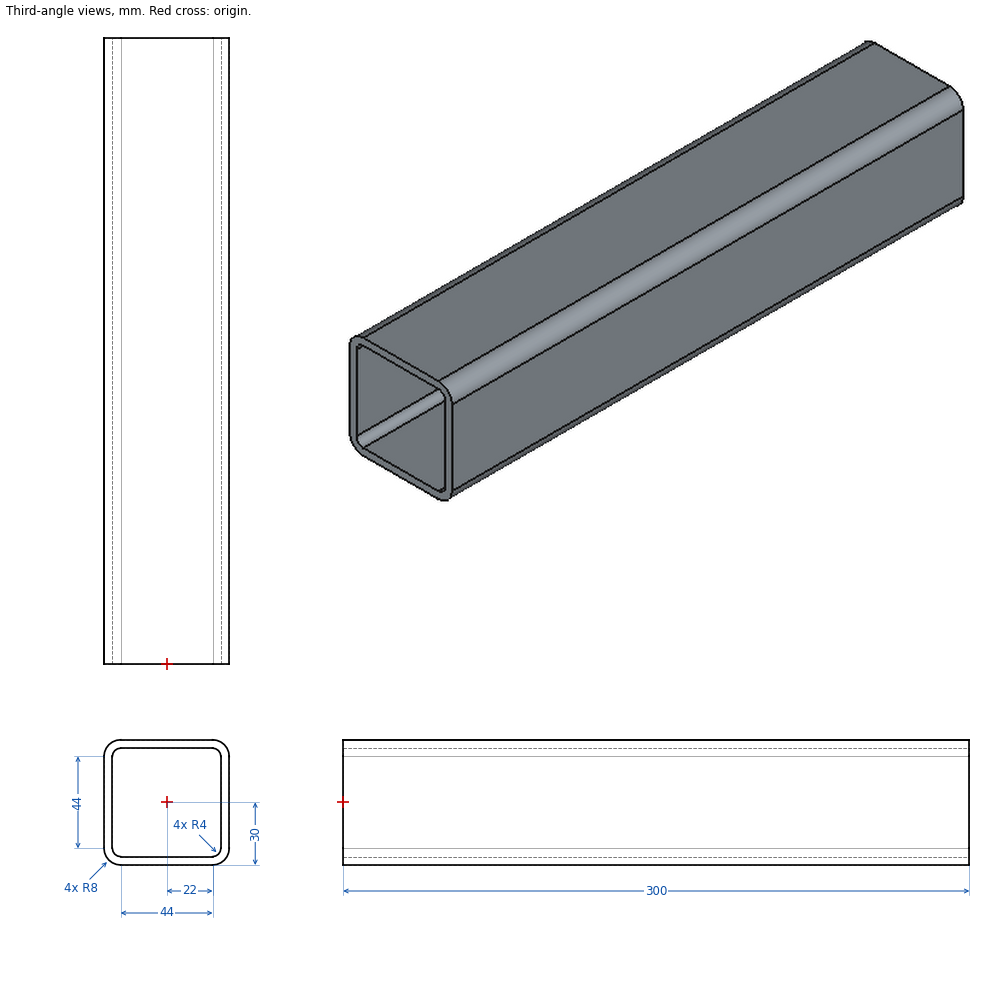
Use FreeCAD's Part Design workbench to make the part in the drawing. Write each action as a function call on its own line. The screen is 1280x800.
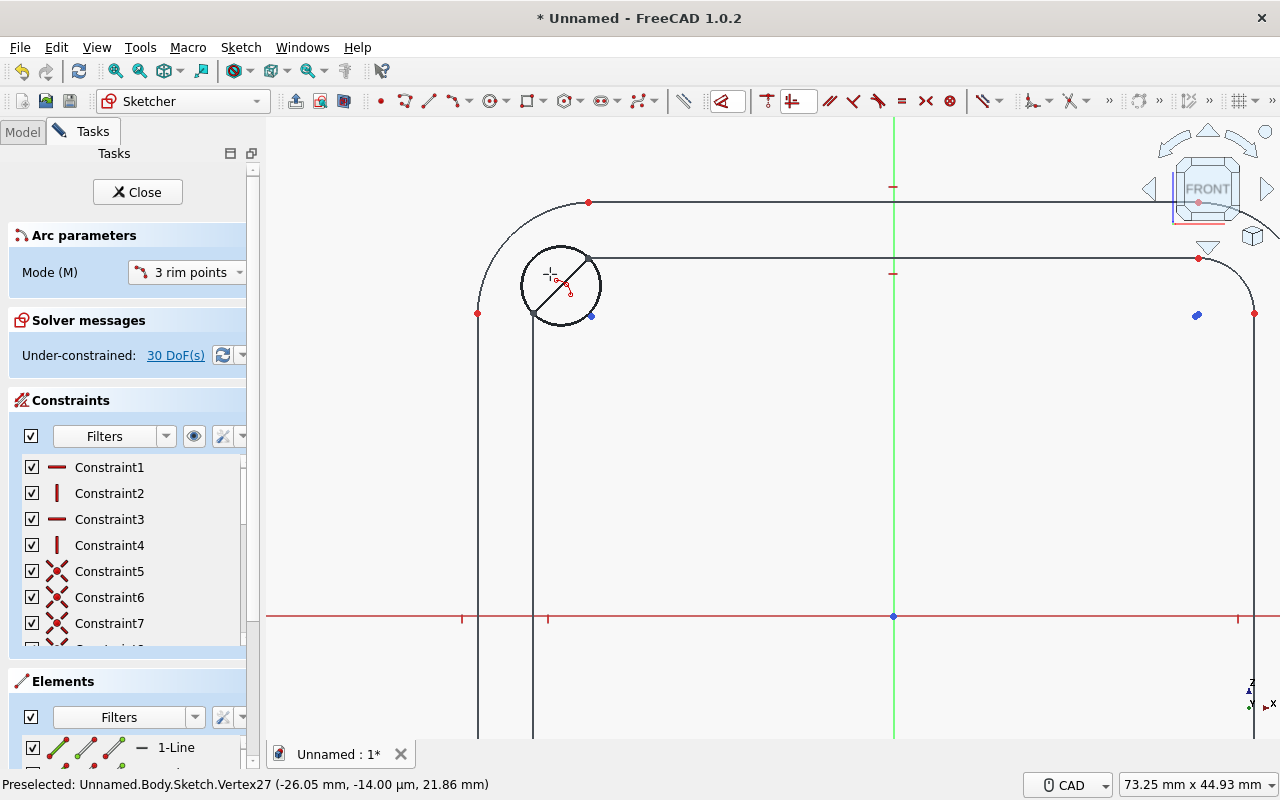
click(550, 273)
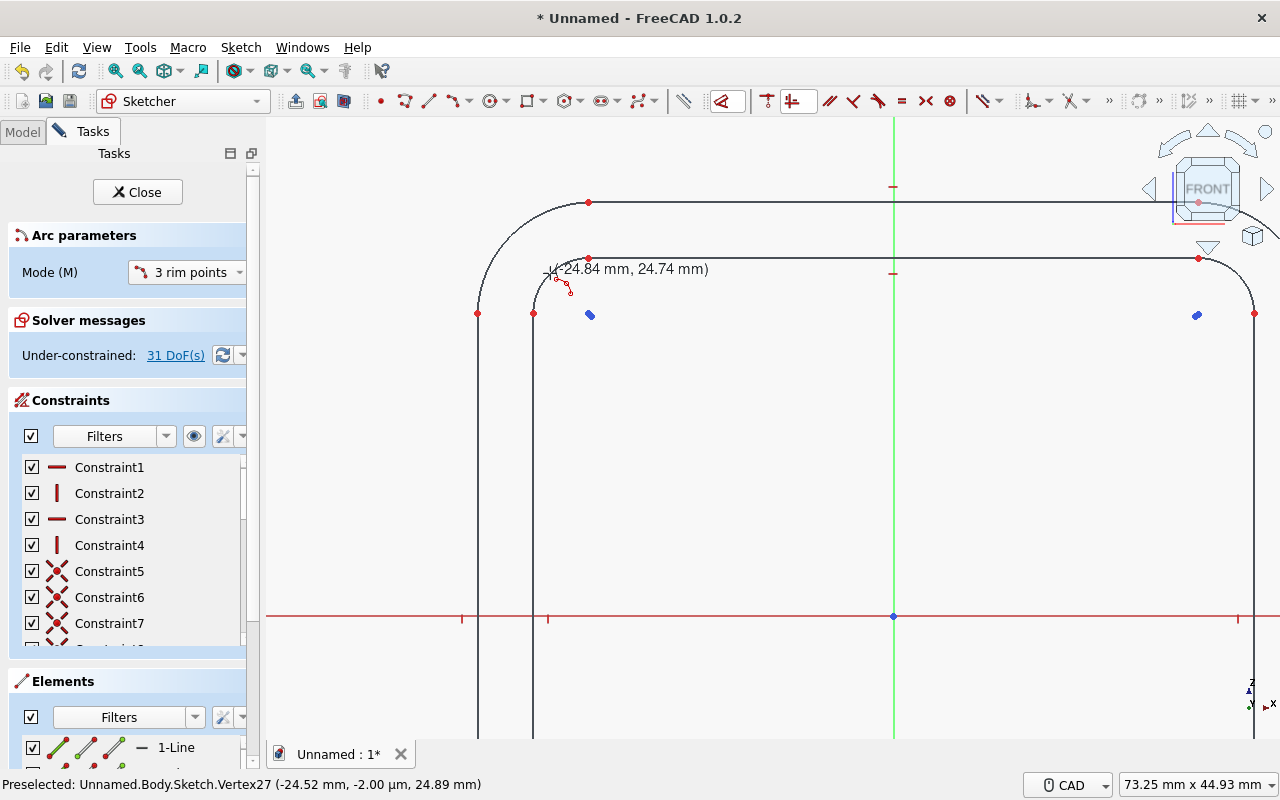
scroll(550, 274, down, 4)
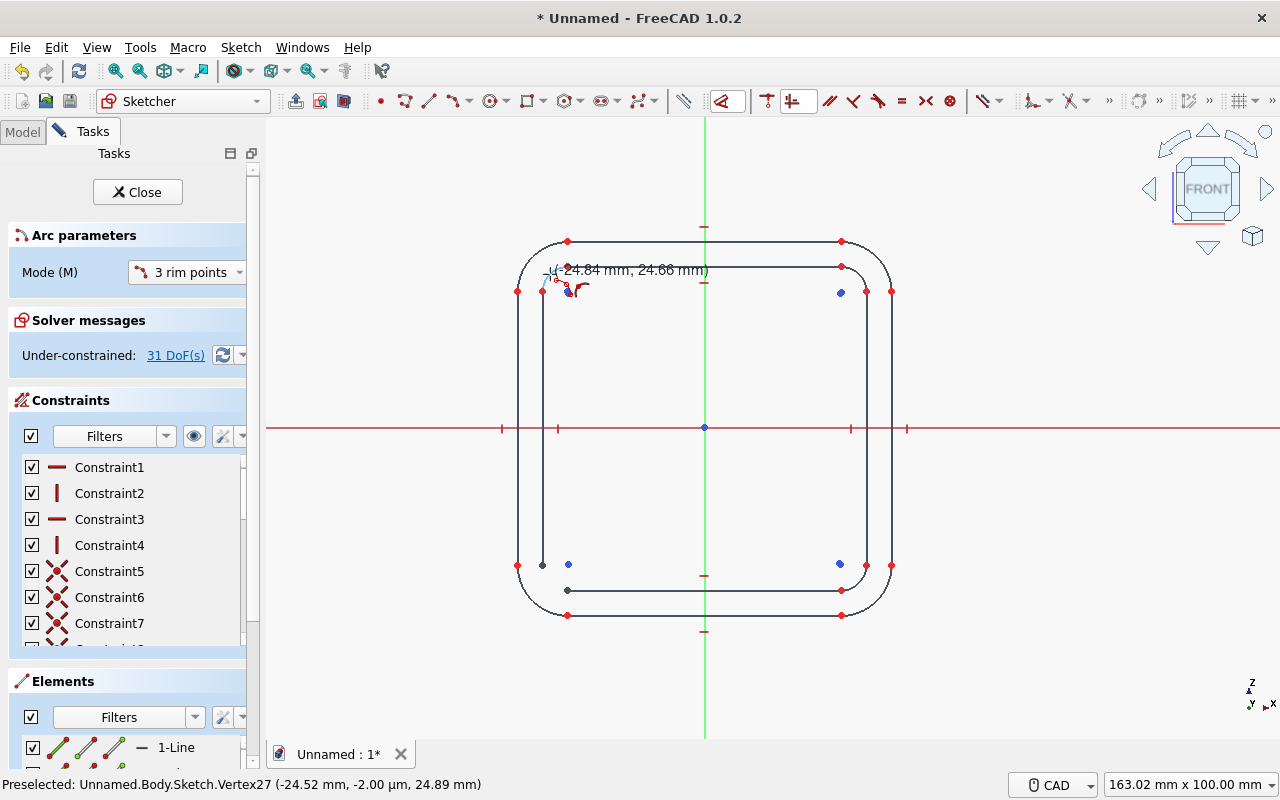
click(543, 566)
click(568, 591)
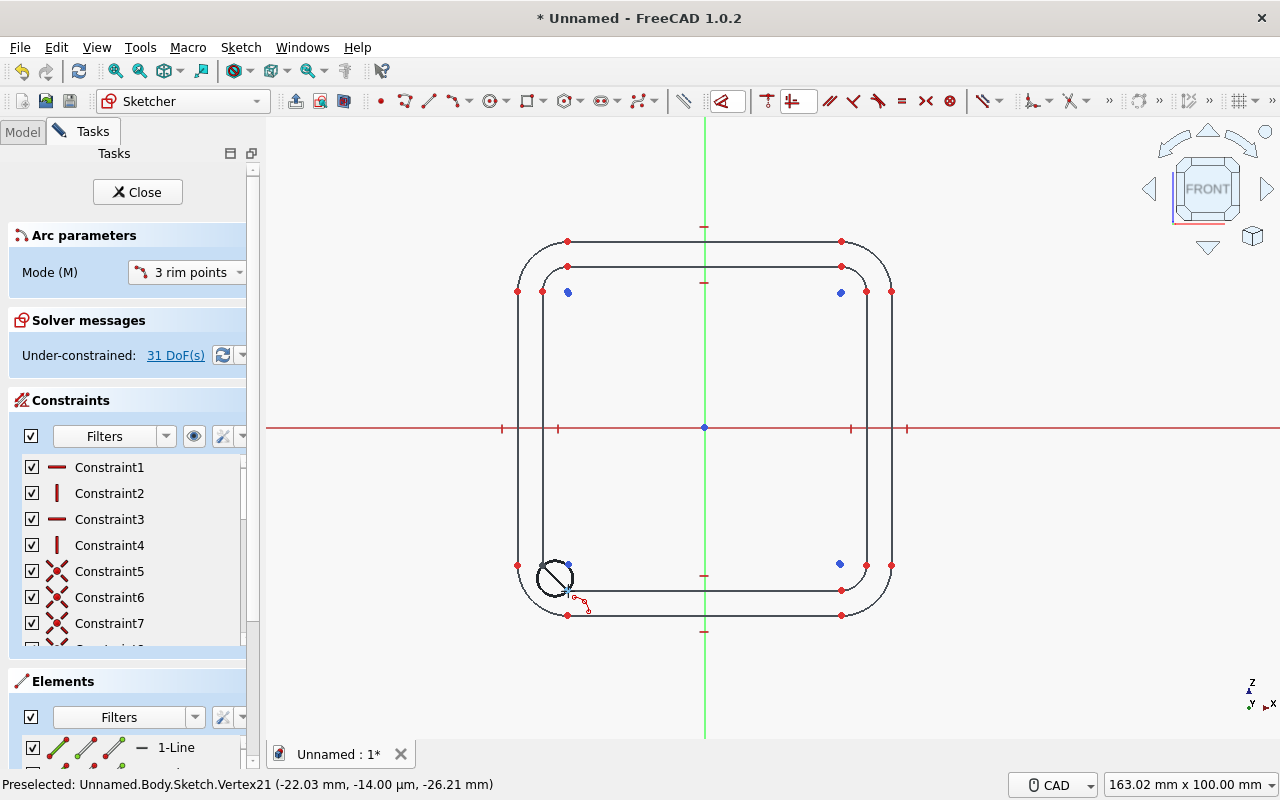
scroll(550, 582, up, 4)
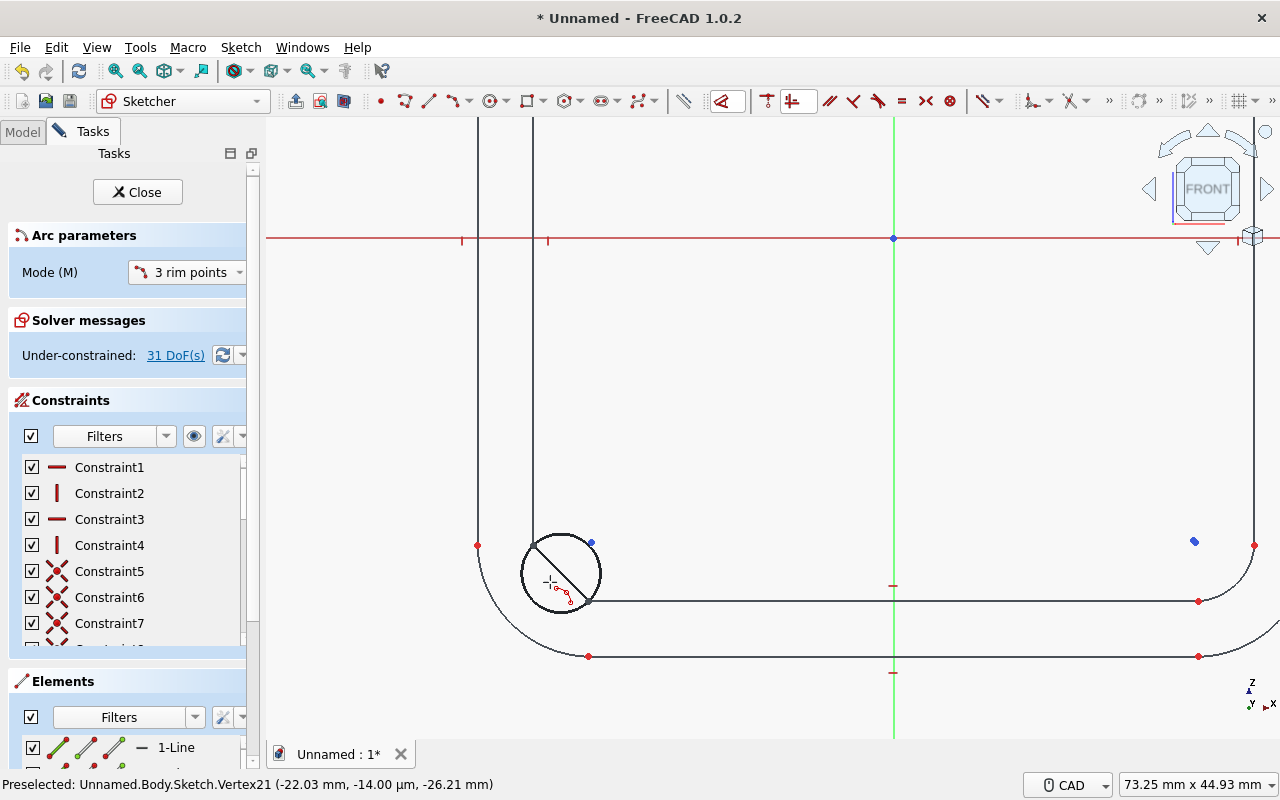
click(550, 582)
key(Escape)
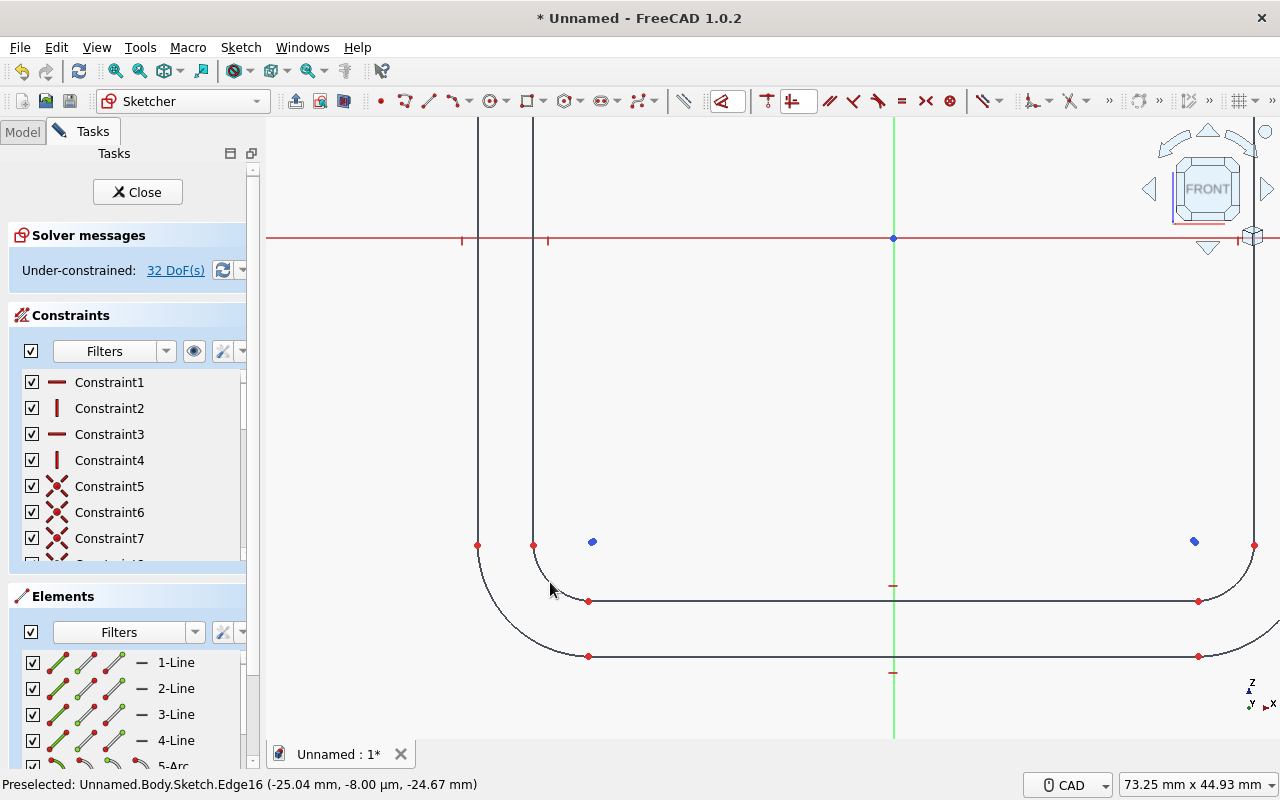
click(1016, 657)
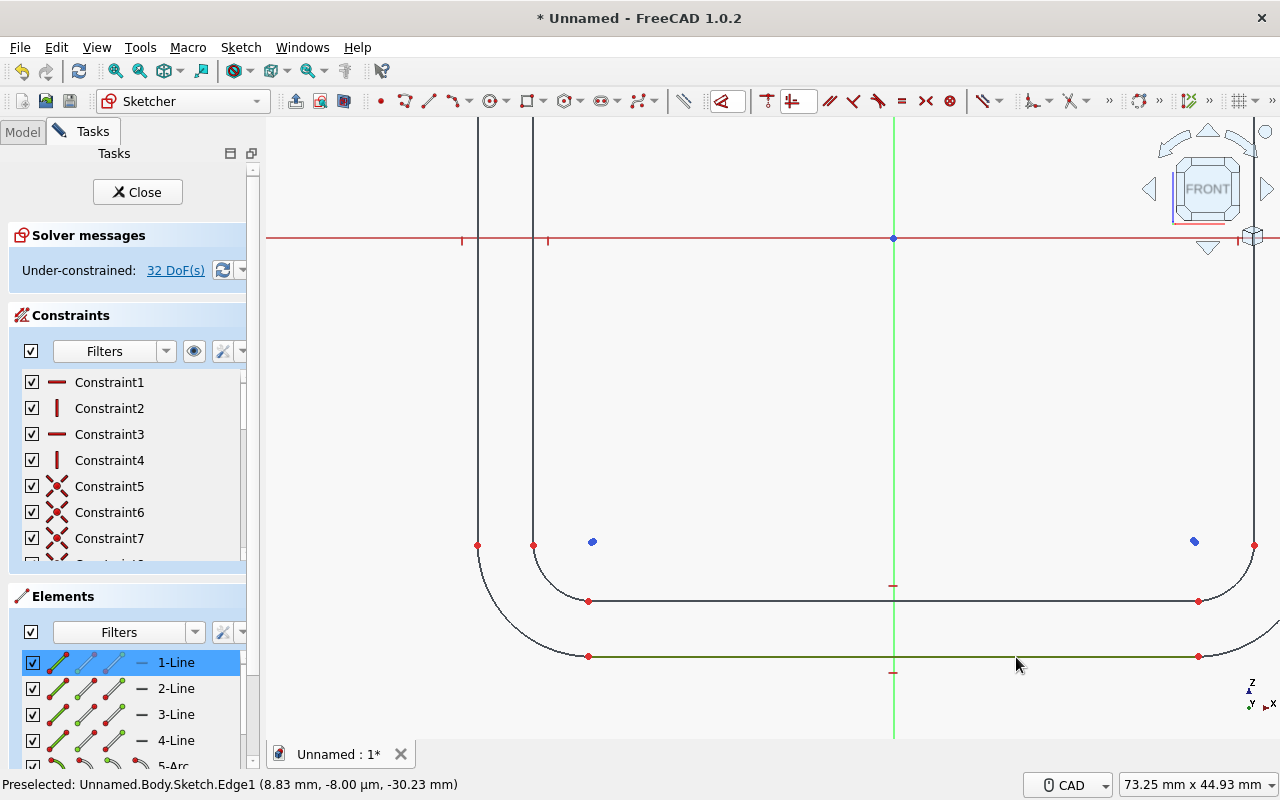
click(491, 595)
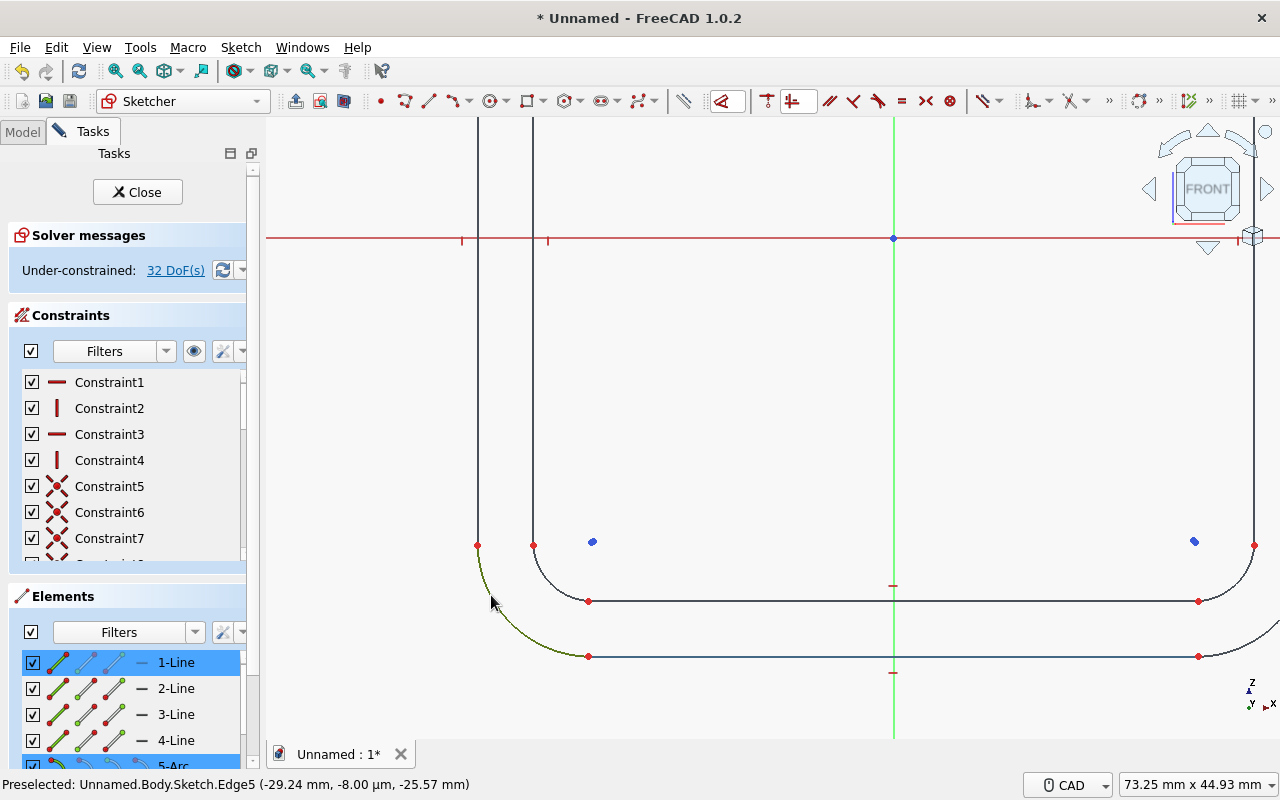
key(t)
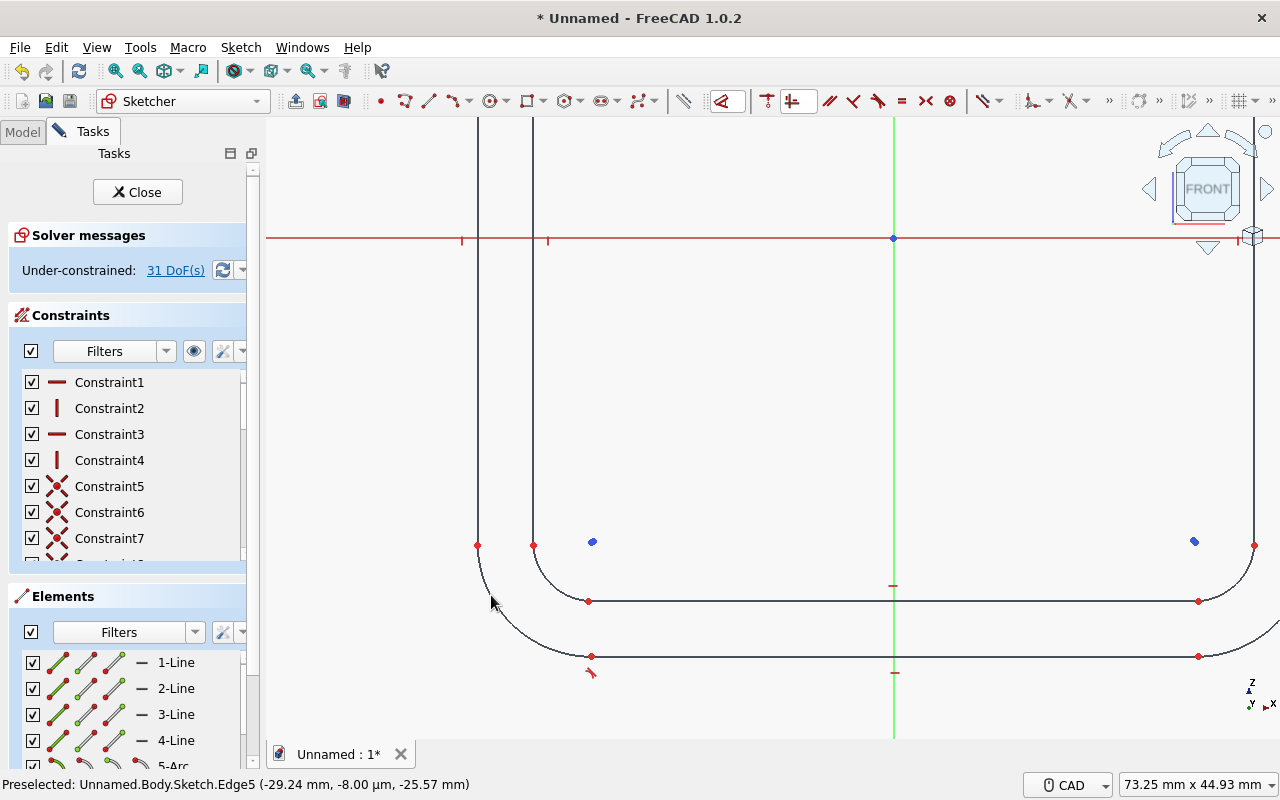
click(1017, 657)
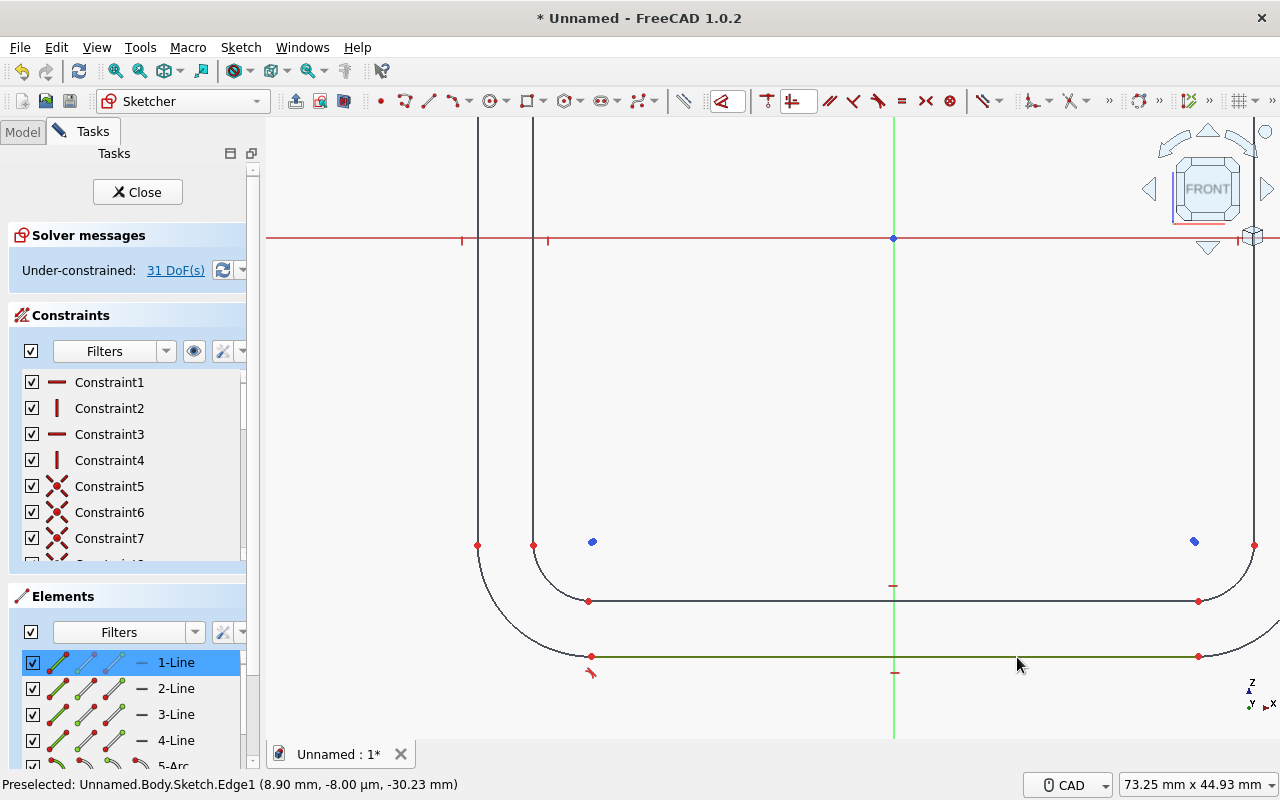
scroll(550, 583, down, 4)